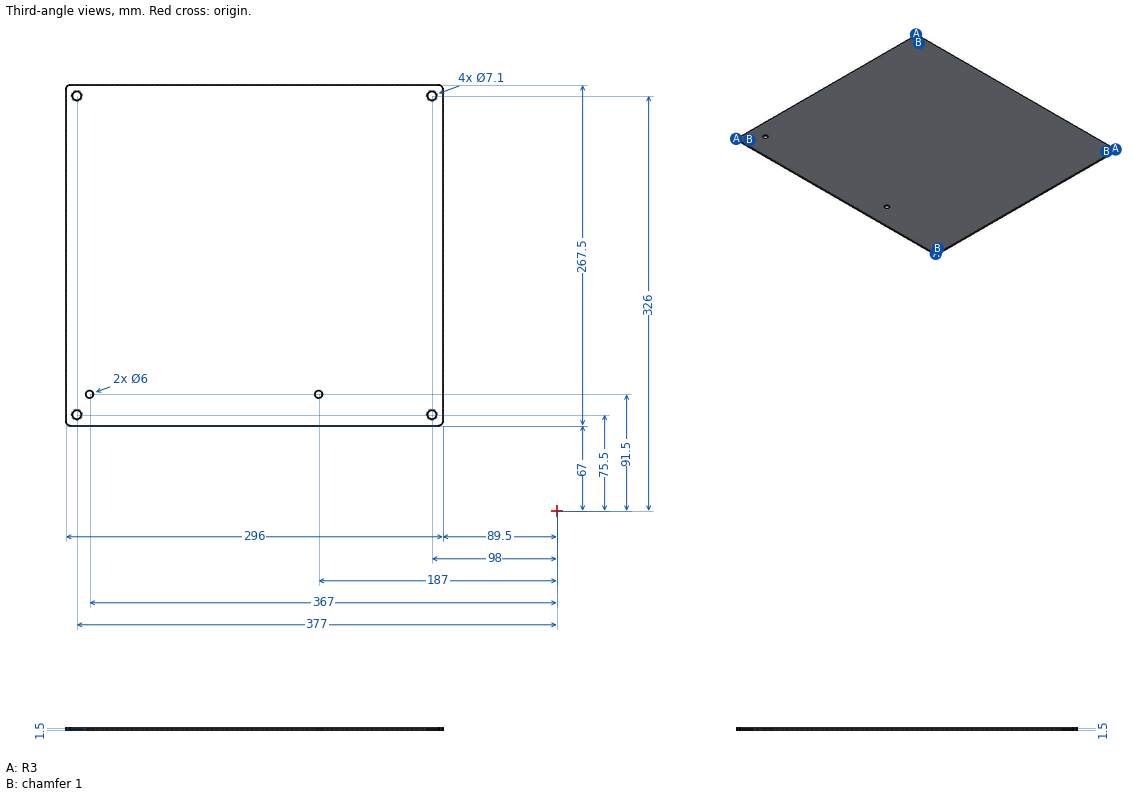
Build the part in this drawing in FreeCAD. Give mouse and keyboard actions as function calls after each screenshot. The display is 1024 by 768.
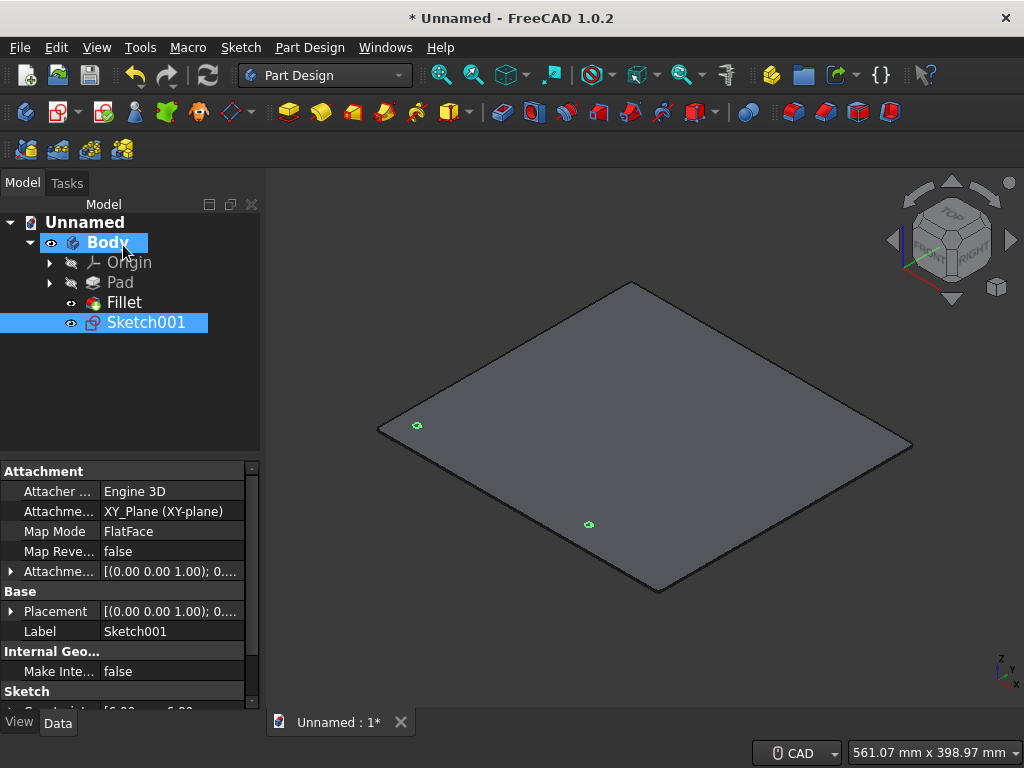
click(504, 112)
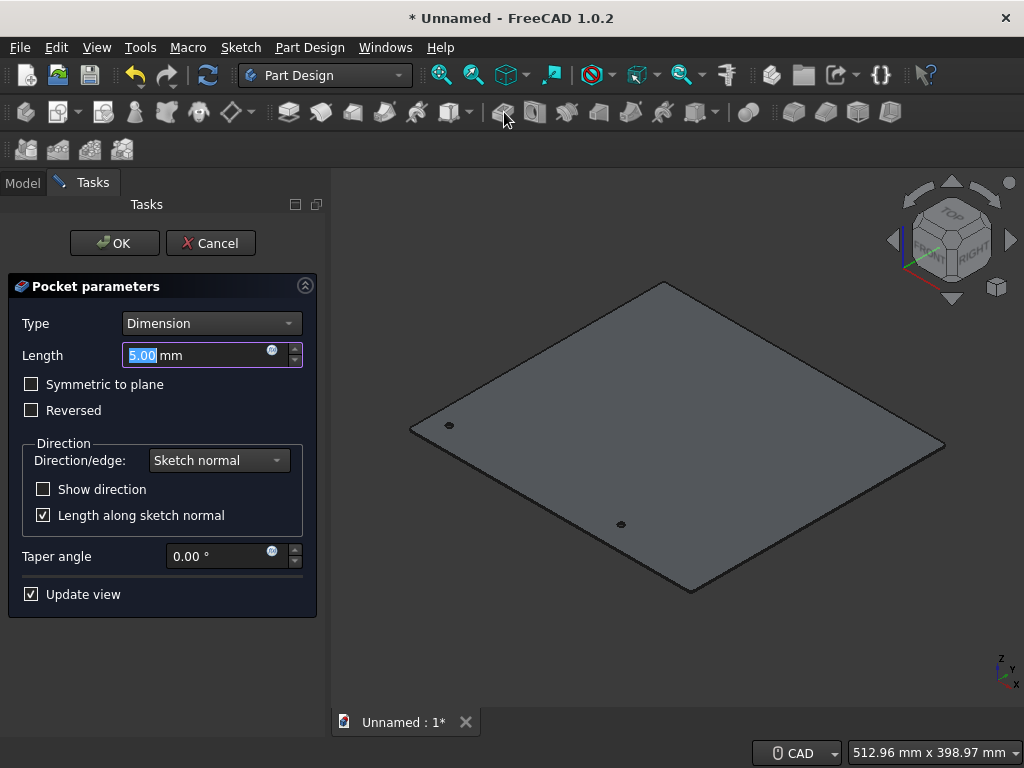
text(1.5)
key(Tab)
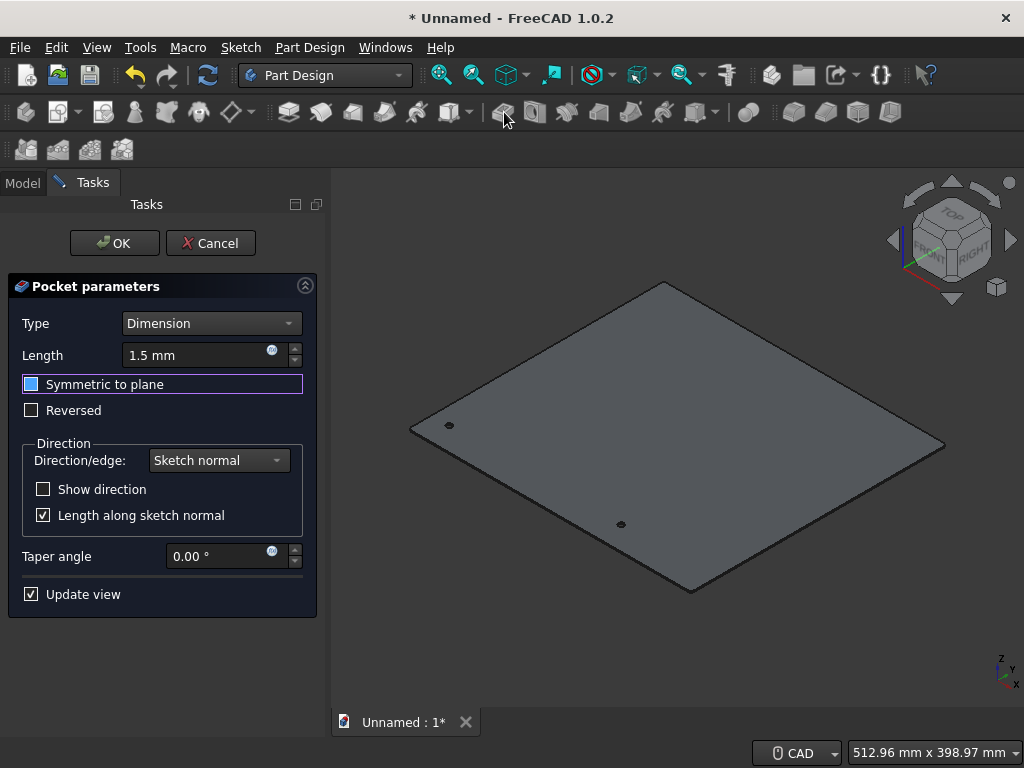
click(115, 243)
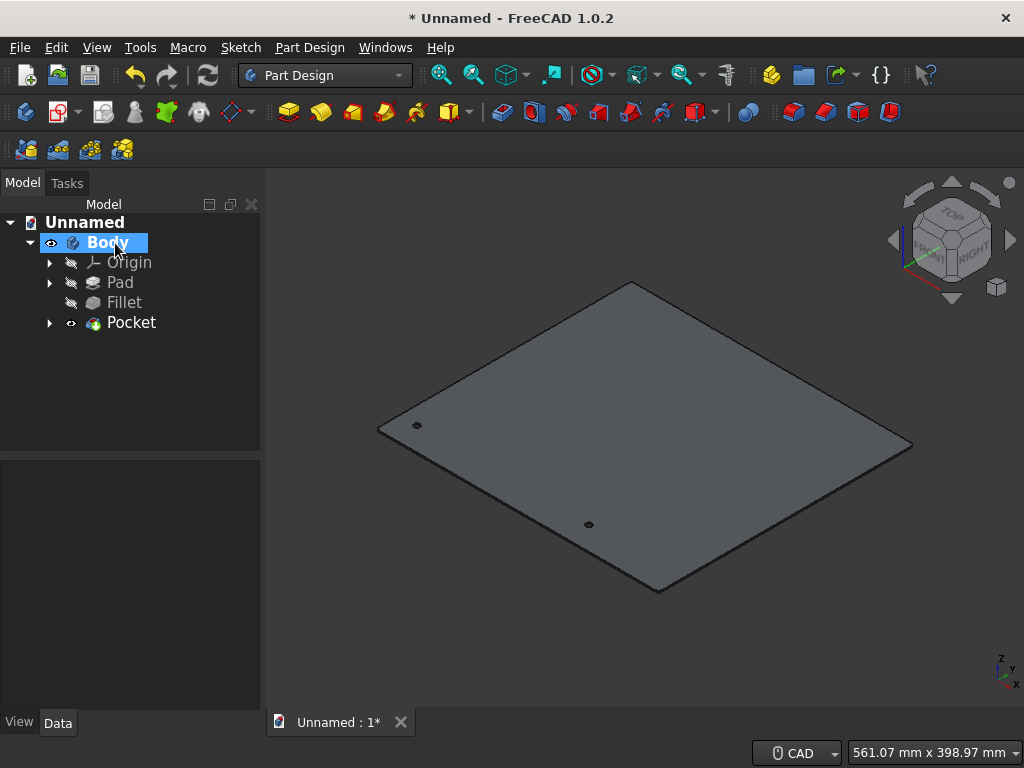
key(5)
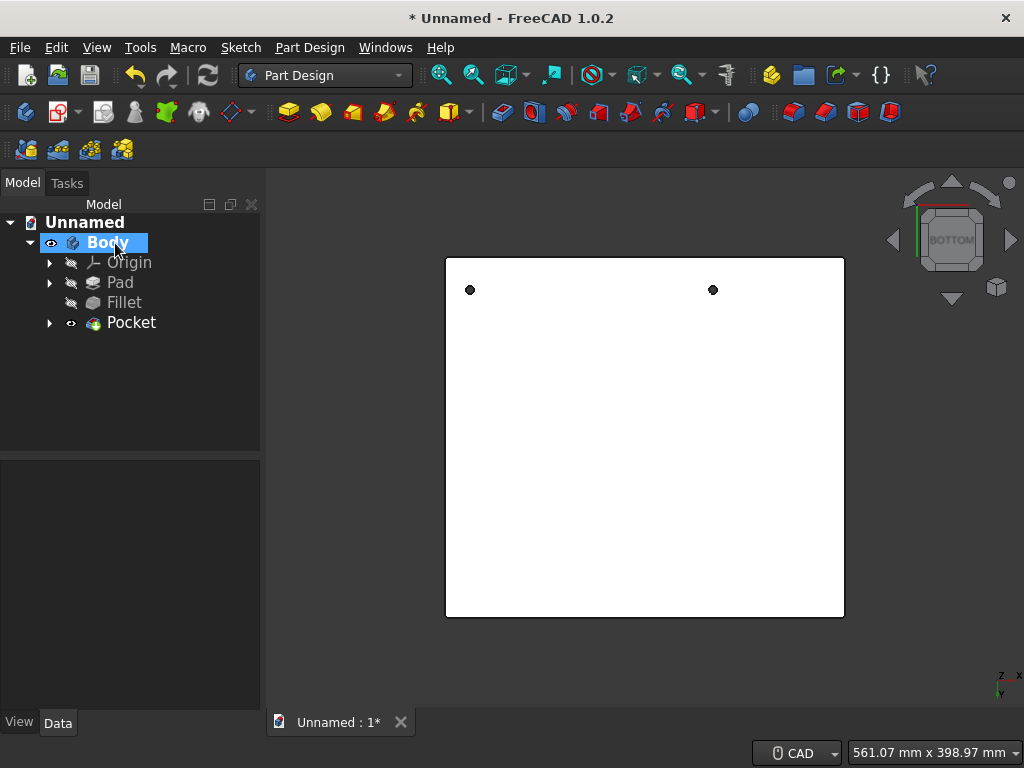
click(645, 437)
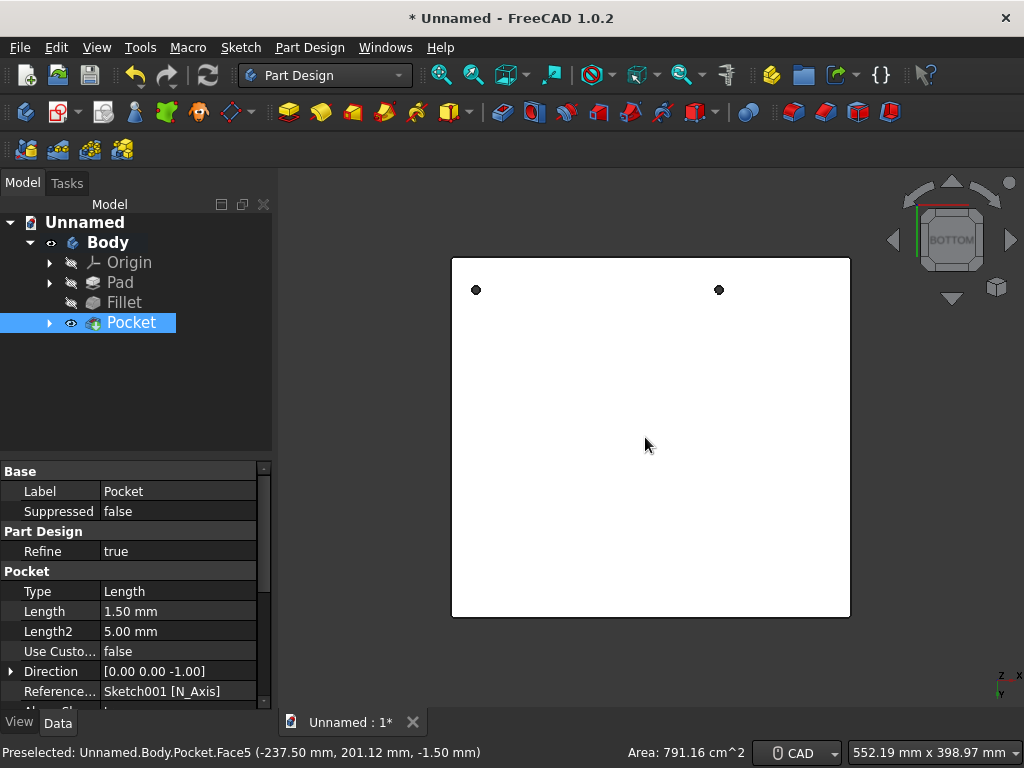
click(58, 112)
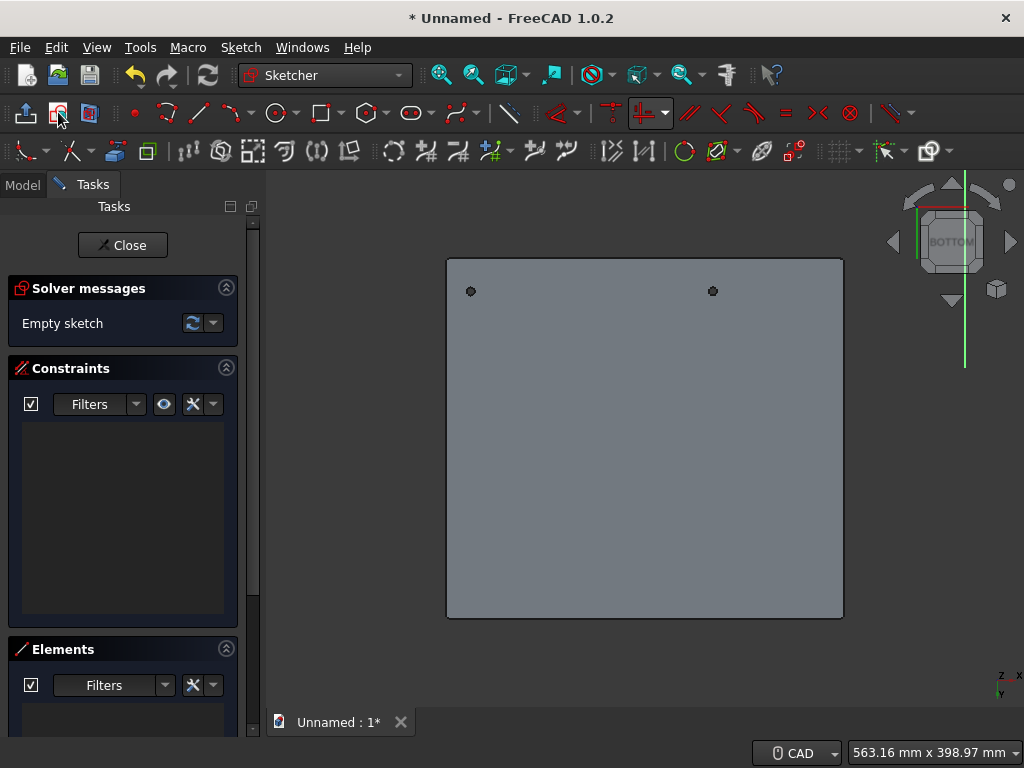
scroll(308, 537, down, 2)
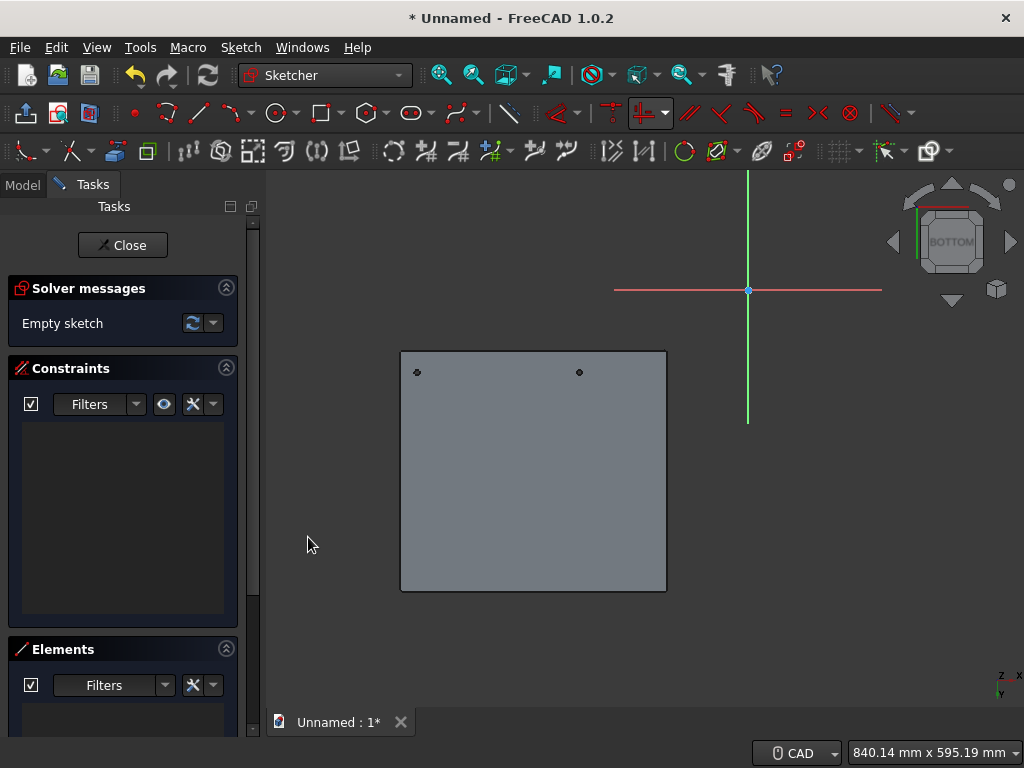
click(276, 114)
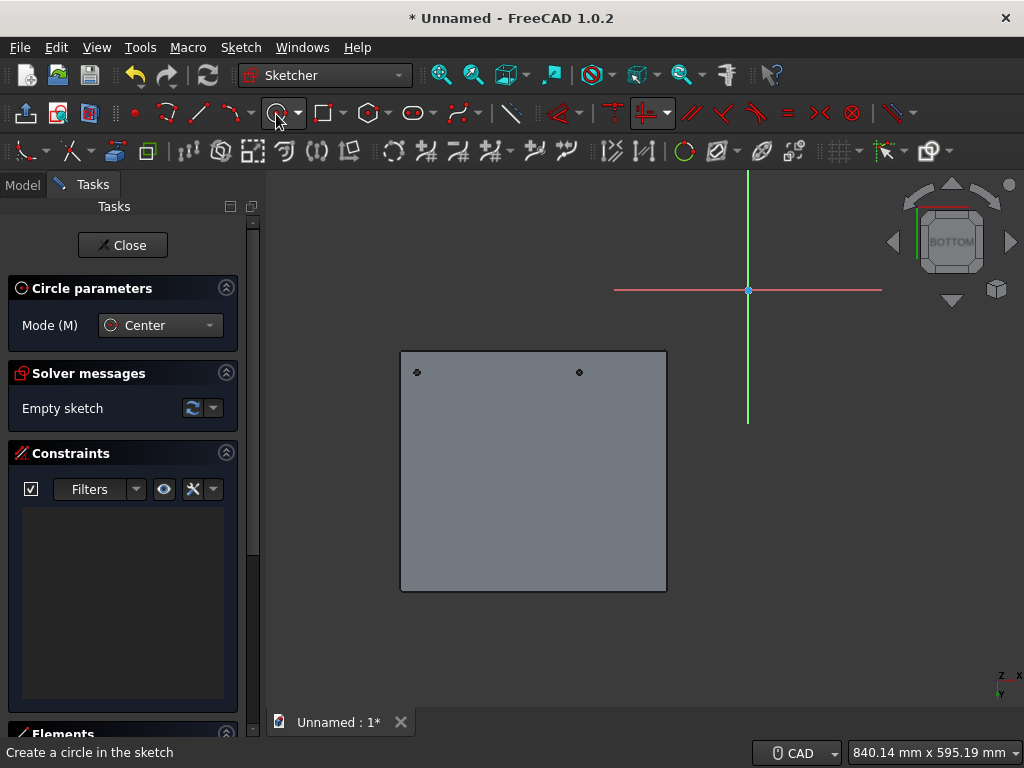
scroll(660, 584, up, 10)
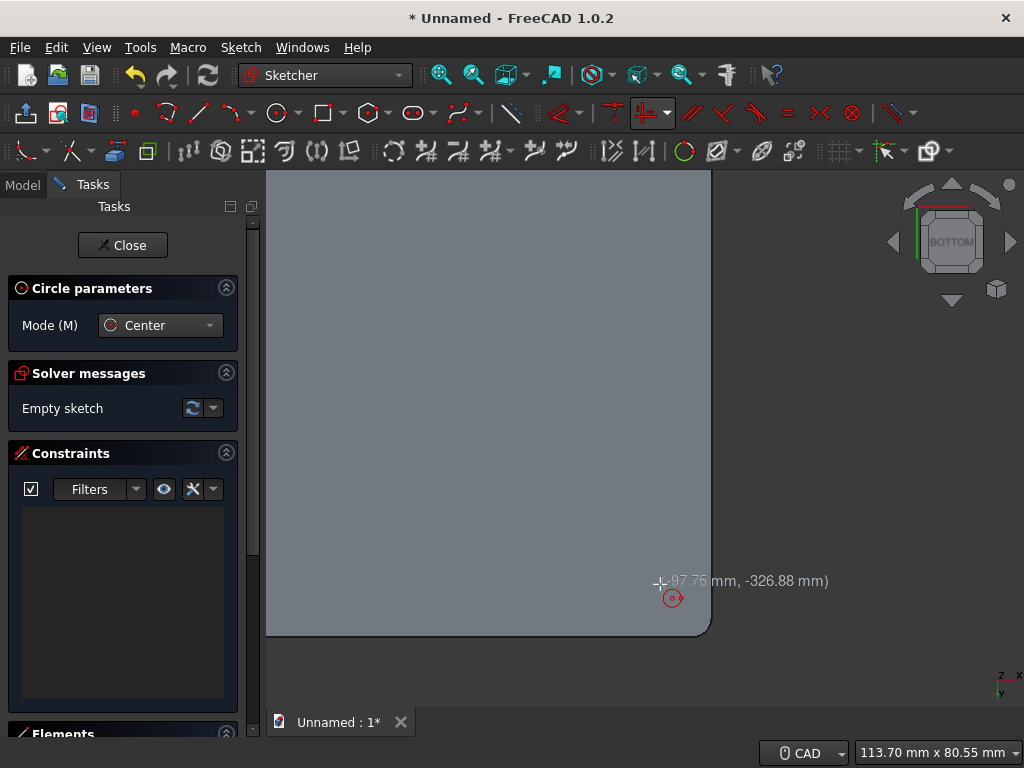
scroll(683, 623, down, 9)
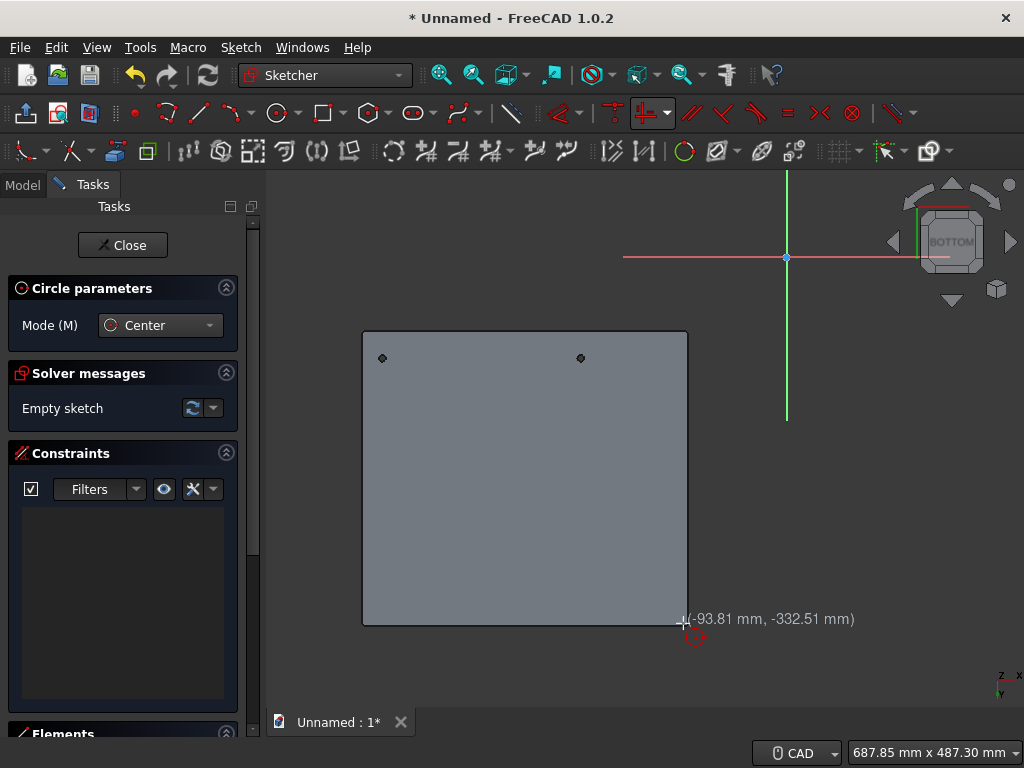
click(679, 617)
move(682, 614)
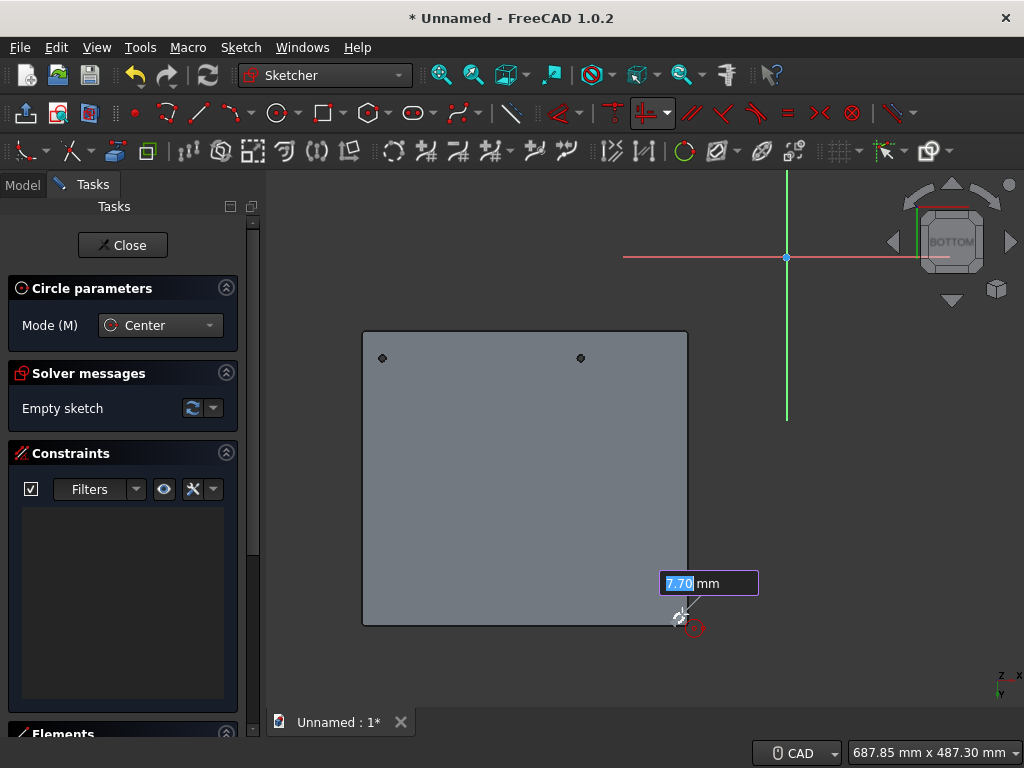
text(7.1)
key(Return)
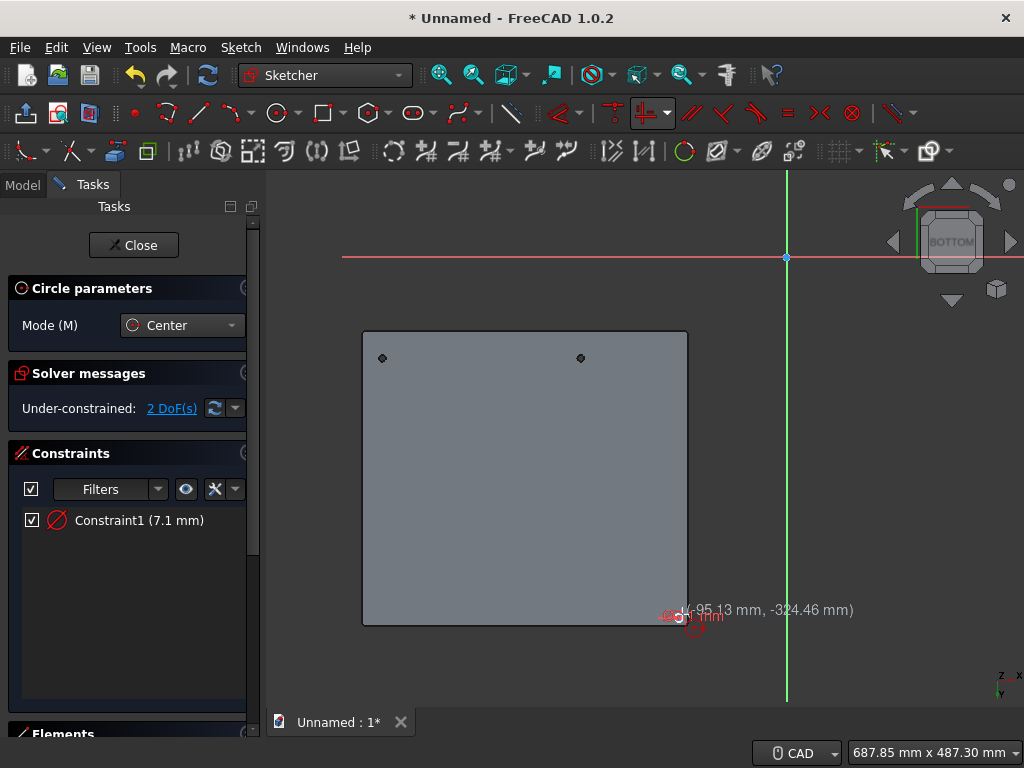
scroll(371, 617, up, 9)